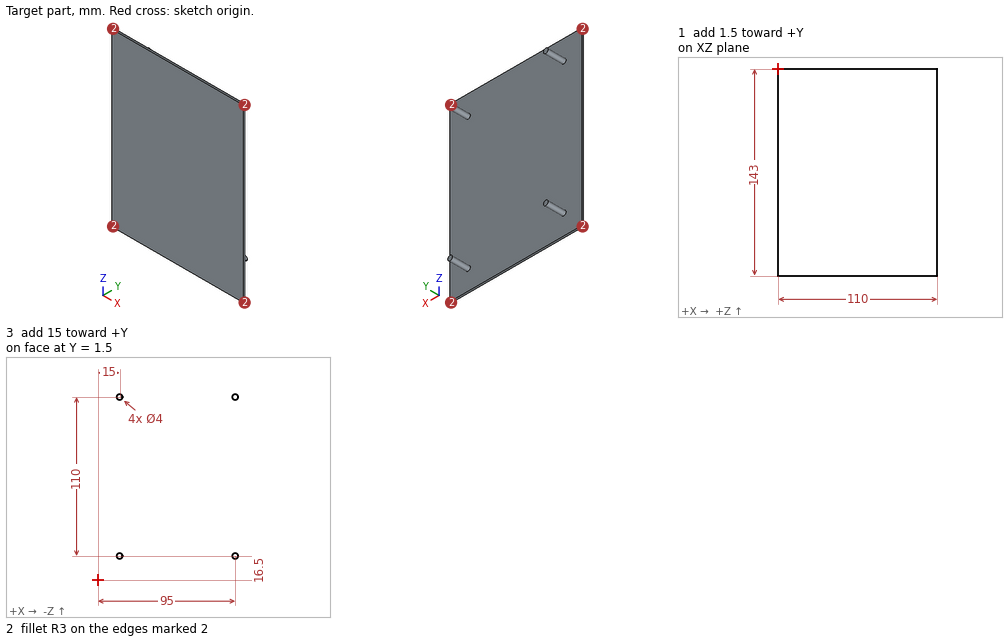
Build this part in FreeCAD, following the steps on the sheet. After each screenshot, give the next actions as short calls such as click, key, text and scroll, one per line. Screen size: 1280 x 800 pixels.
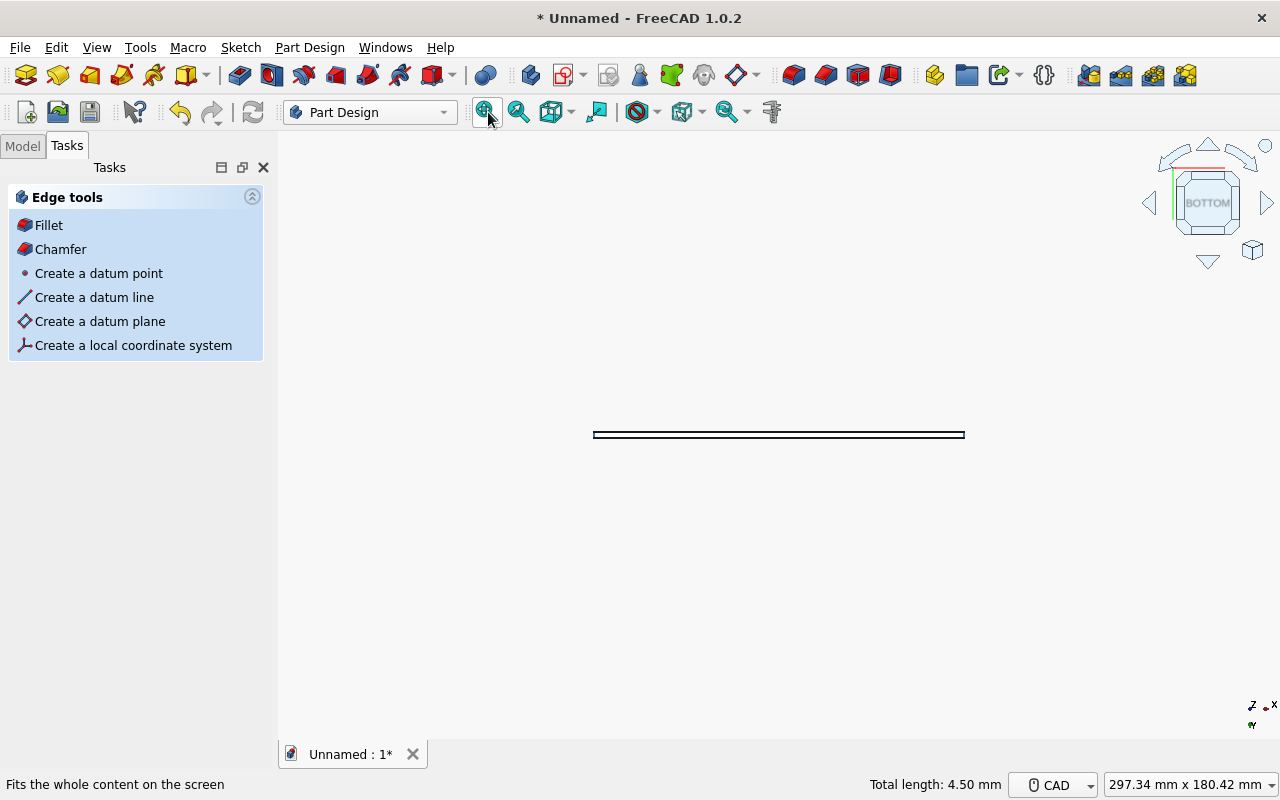
key(4)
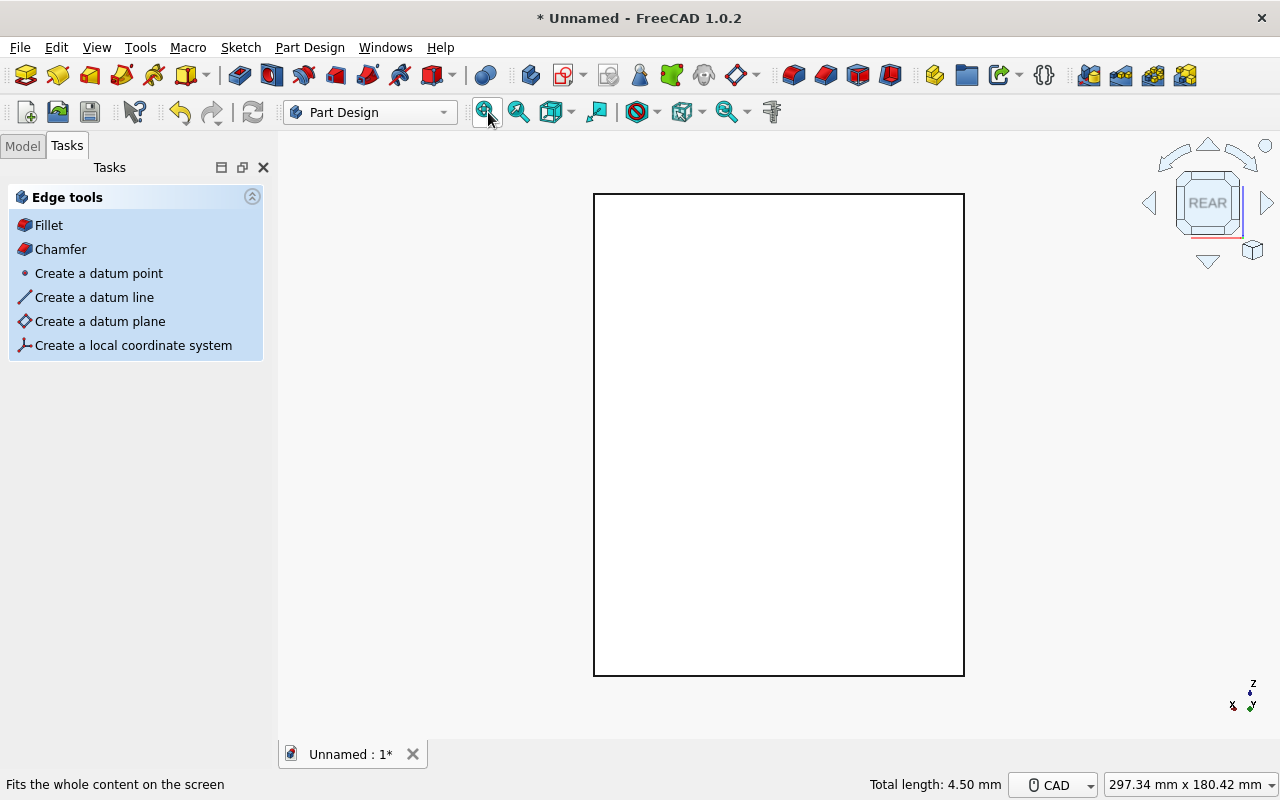
scroll(594, 193, up, 11)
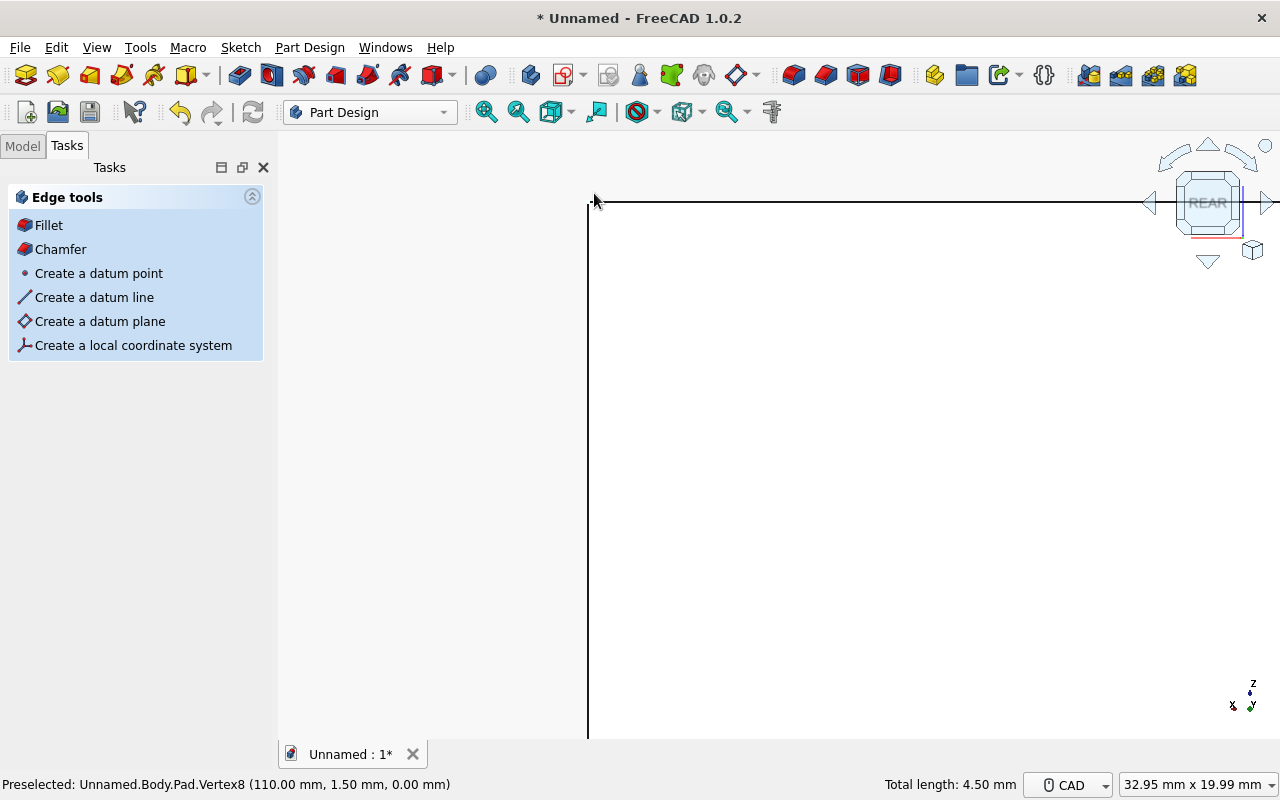
click(488, 112)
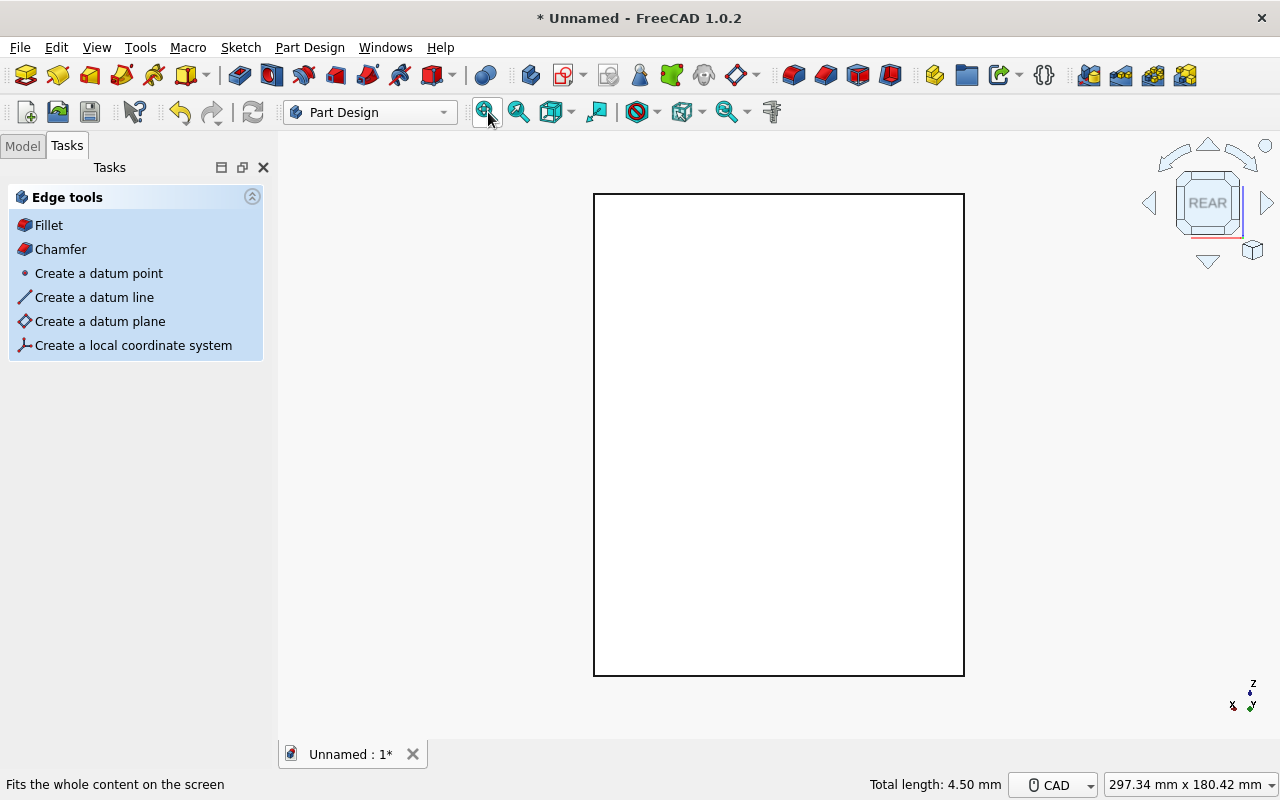
key(6)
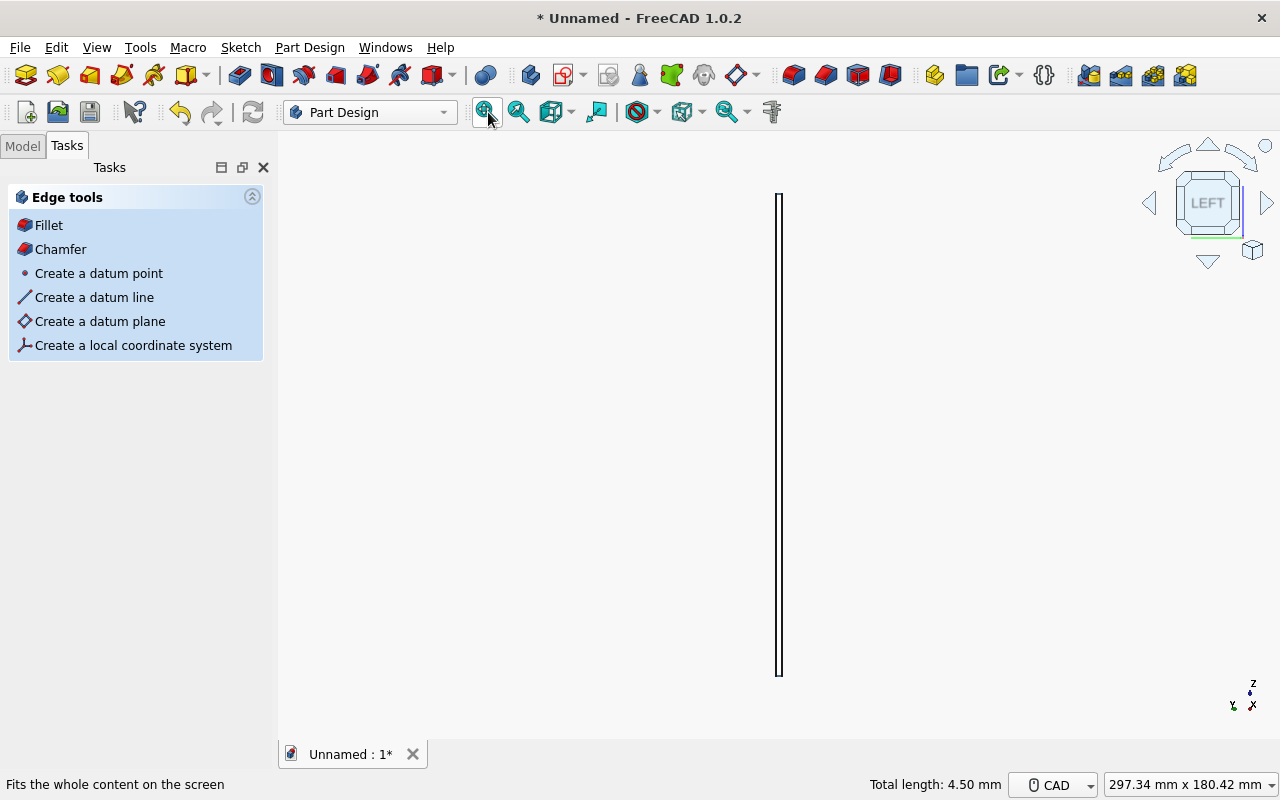
scroll(779, 193, up, 11)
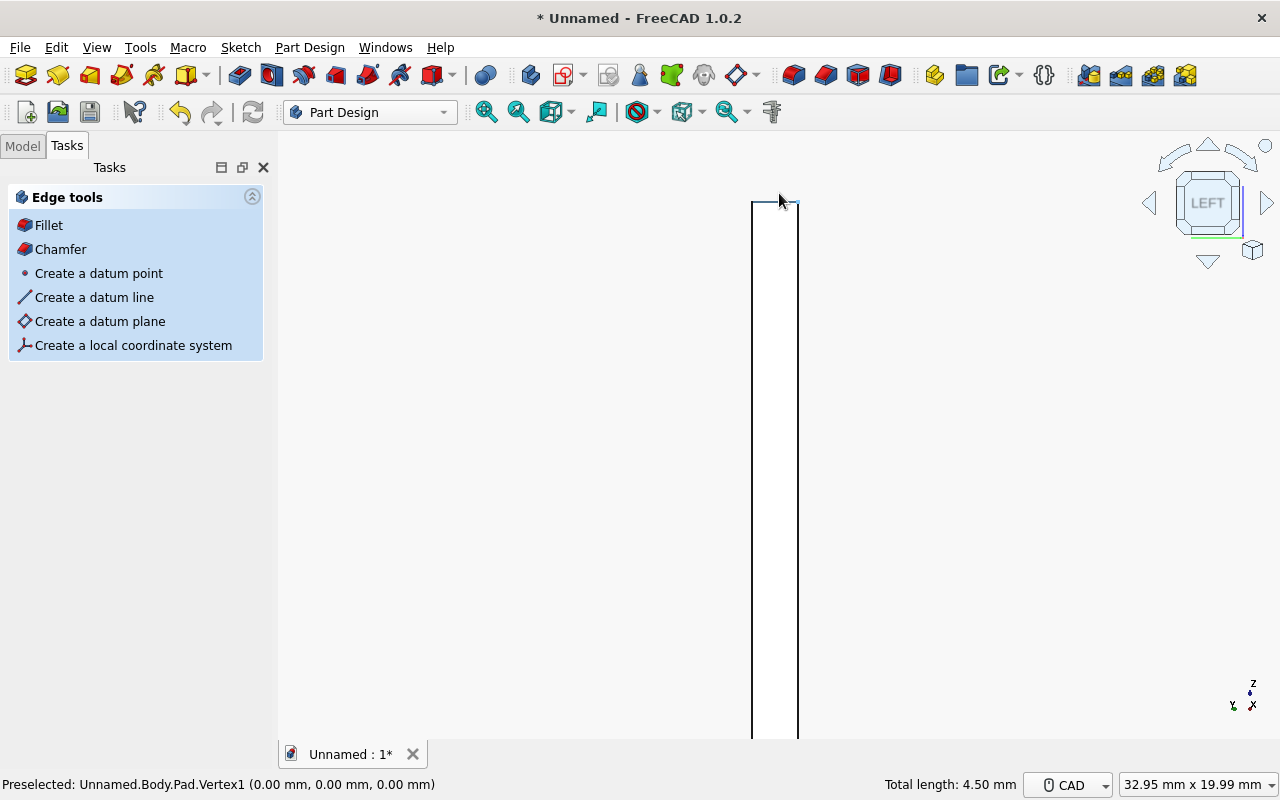
click(488, 112)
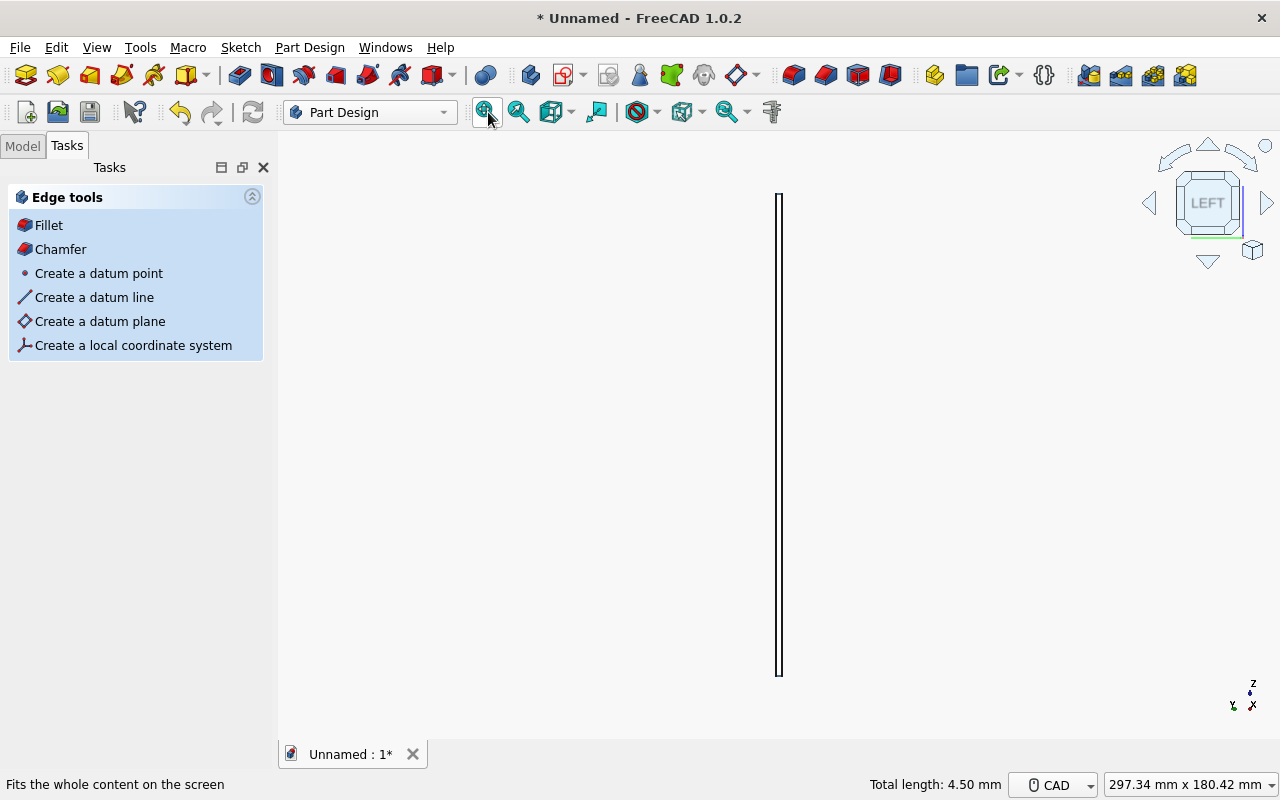
key(v)
key(3)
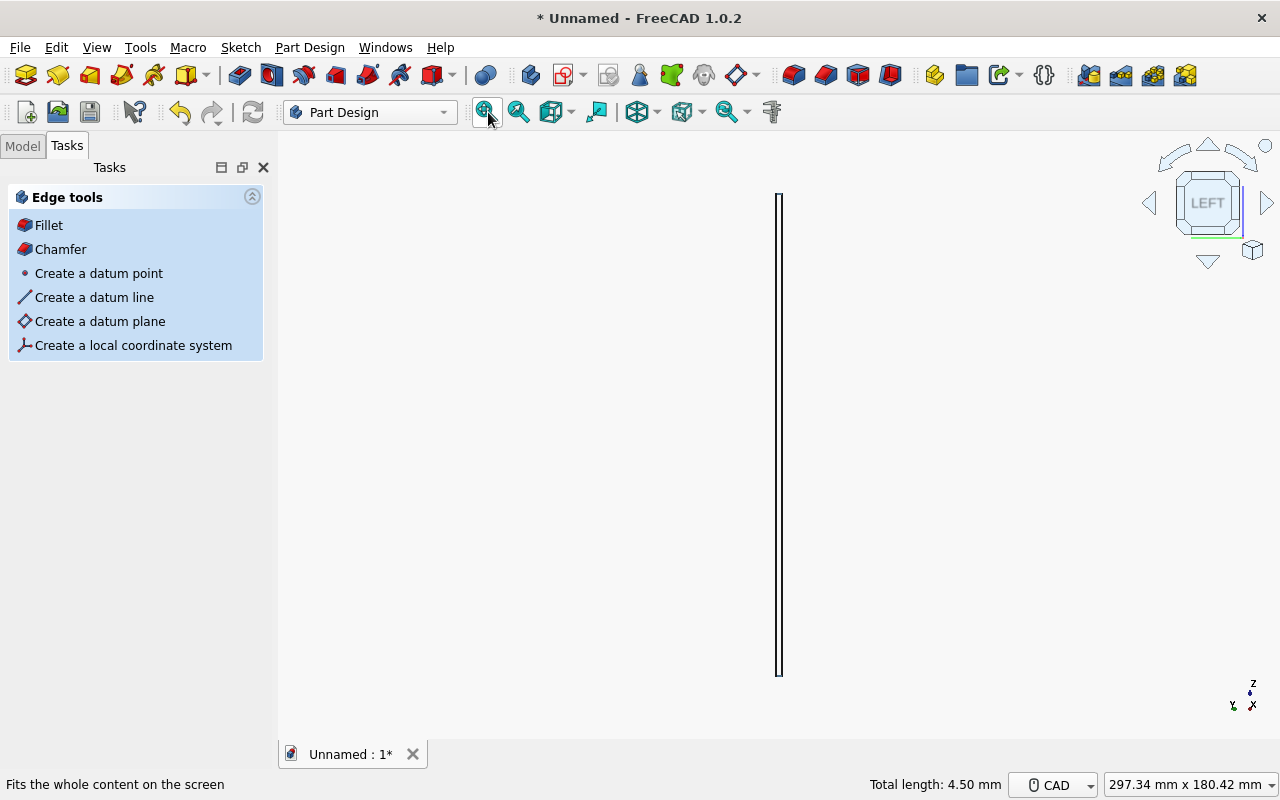
key(0)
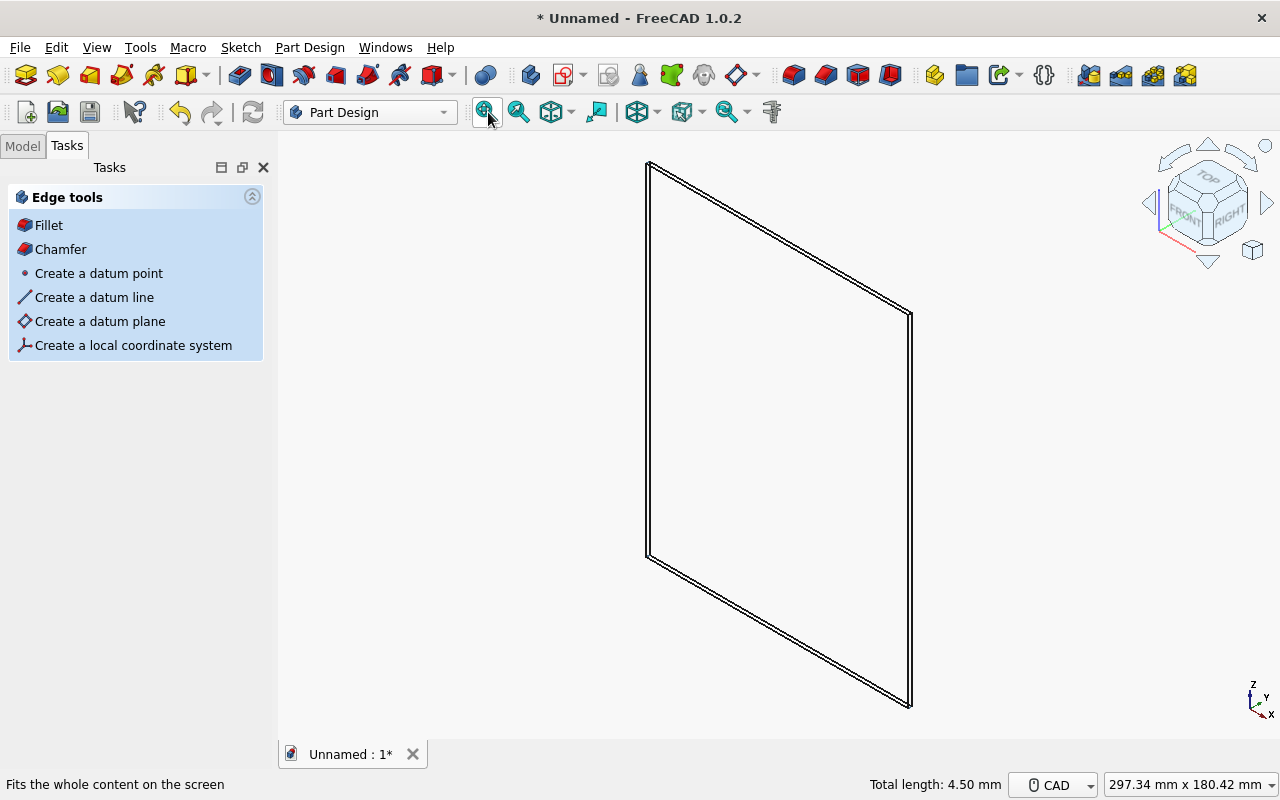
scroll(910, 313, up, 11)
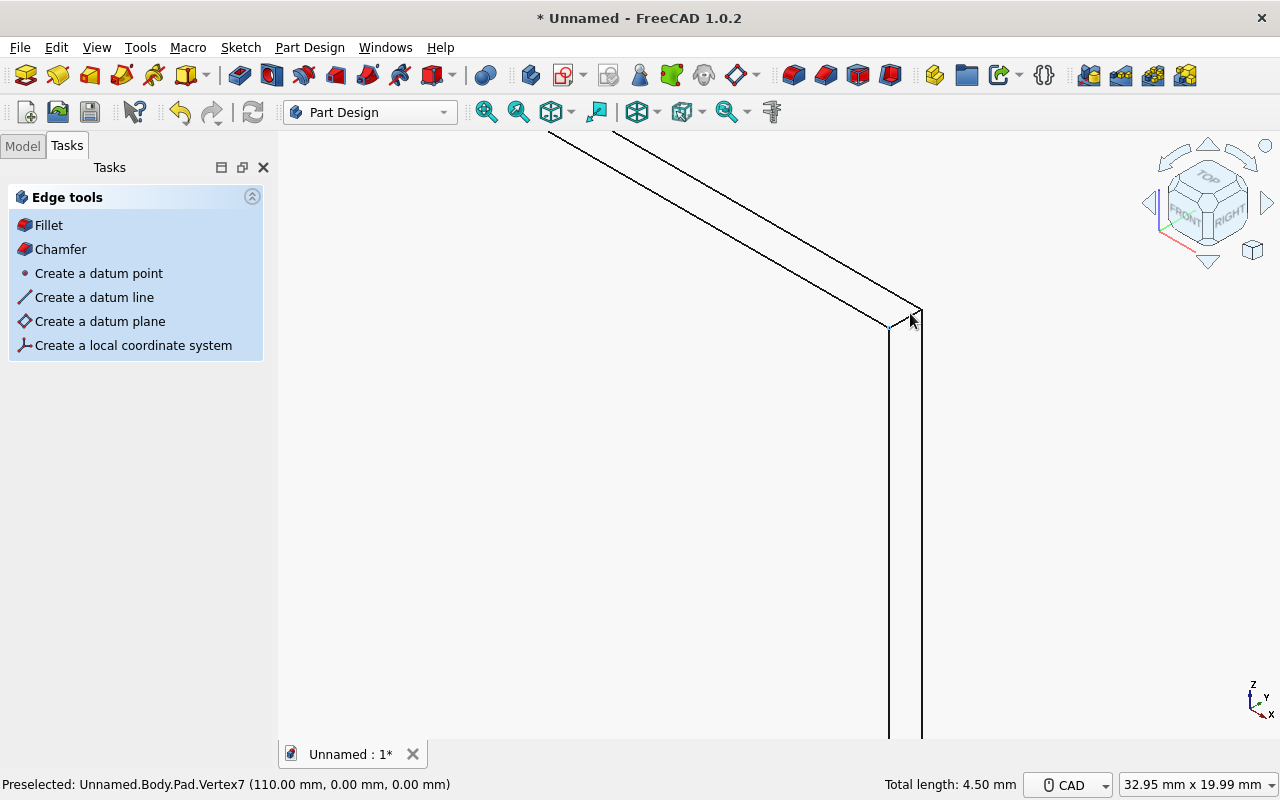
click(905, 318, ctrl)